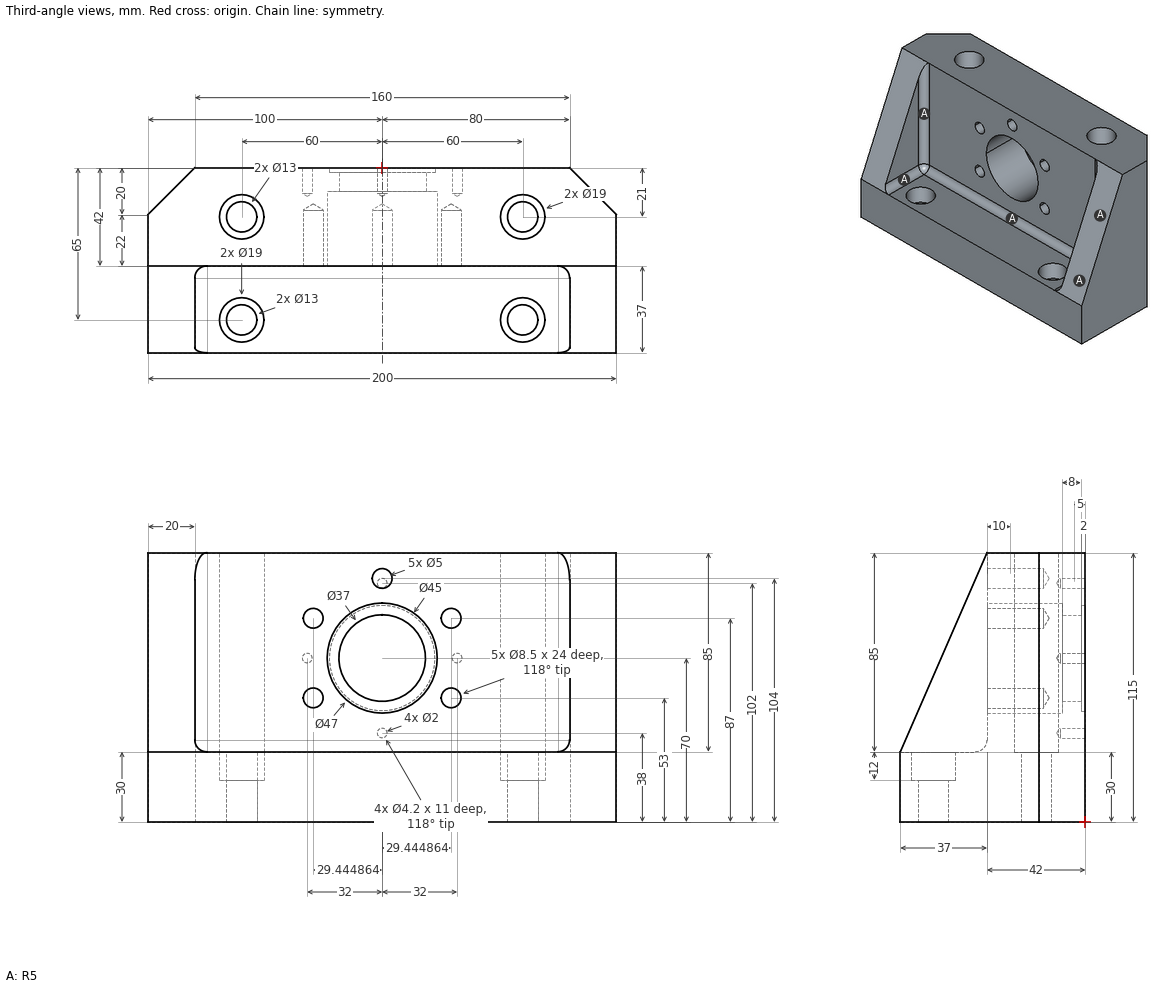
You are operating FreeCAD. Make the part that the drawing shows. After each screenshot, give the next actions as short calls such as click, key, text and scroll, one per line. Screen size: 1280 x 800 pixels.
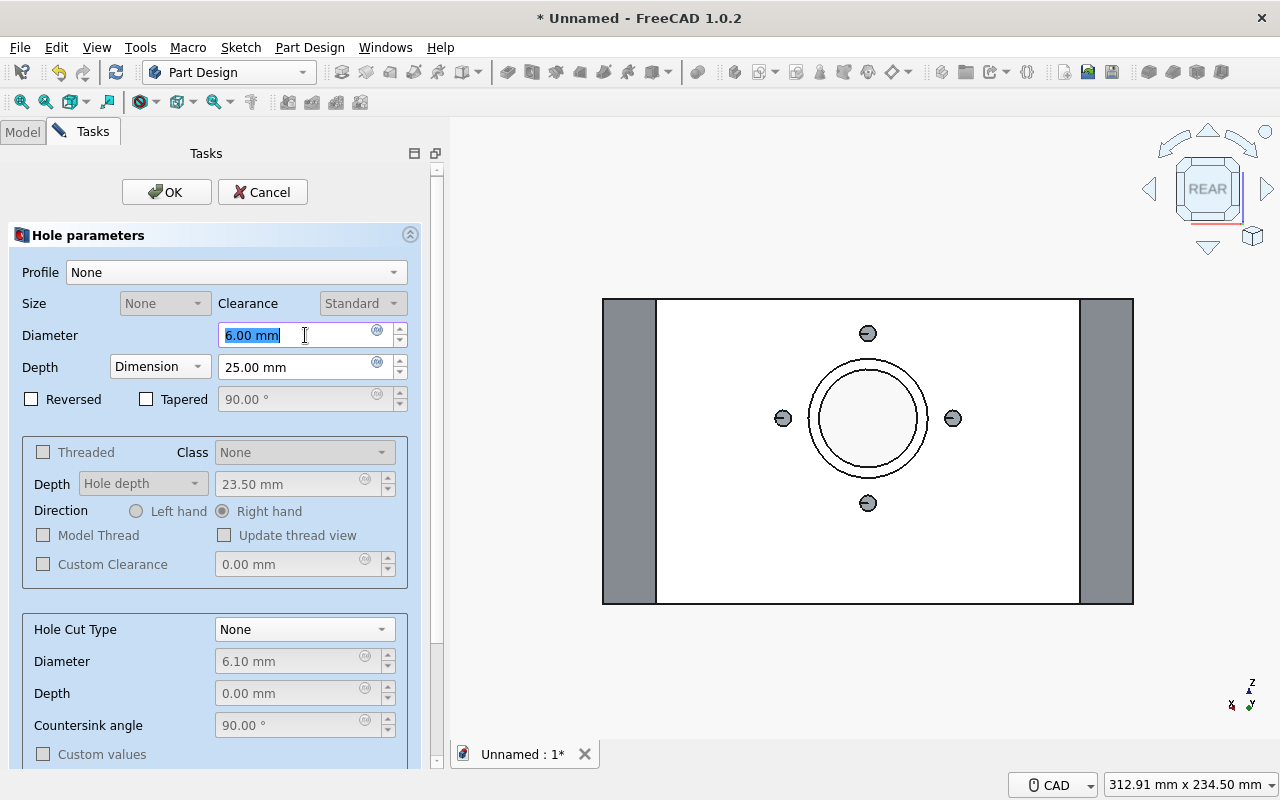
text(4.2)
key(Tab)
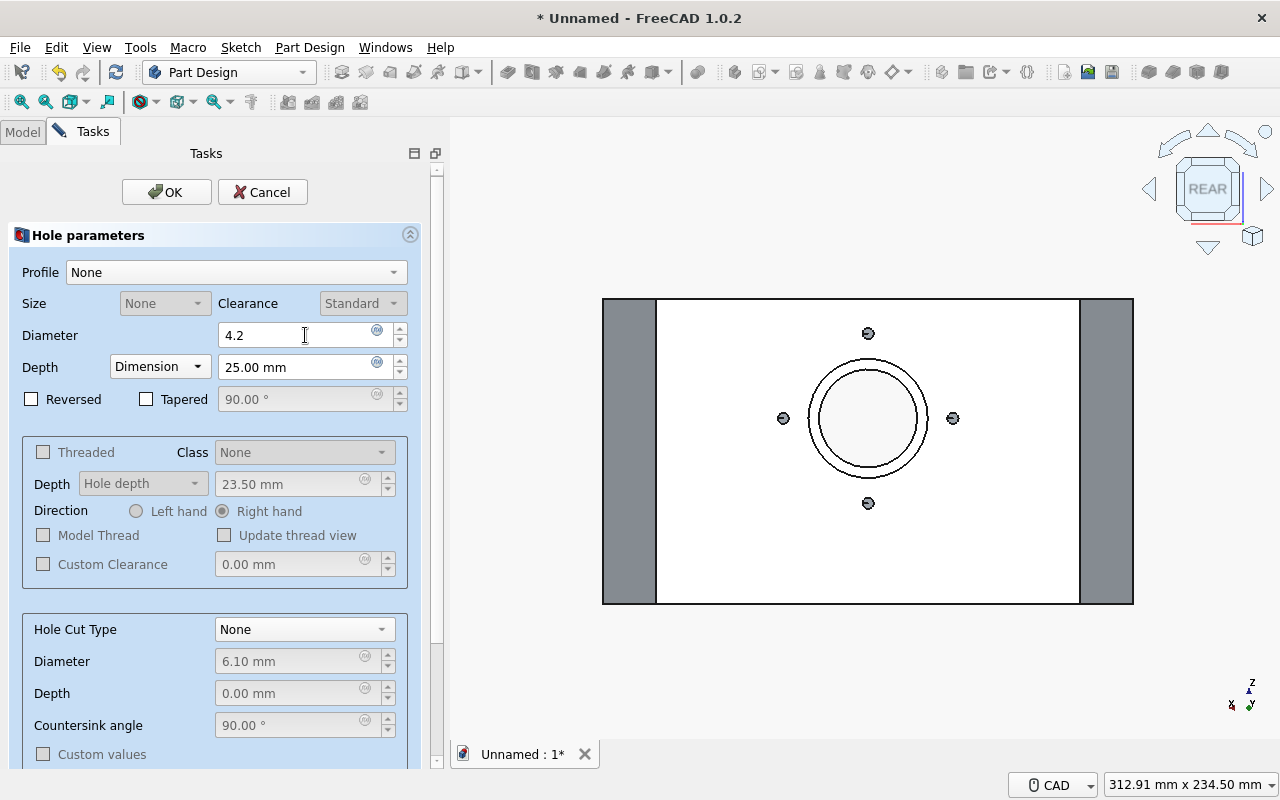
triple_click(305, 367)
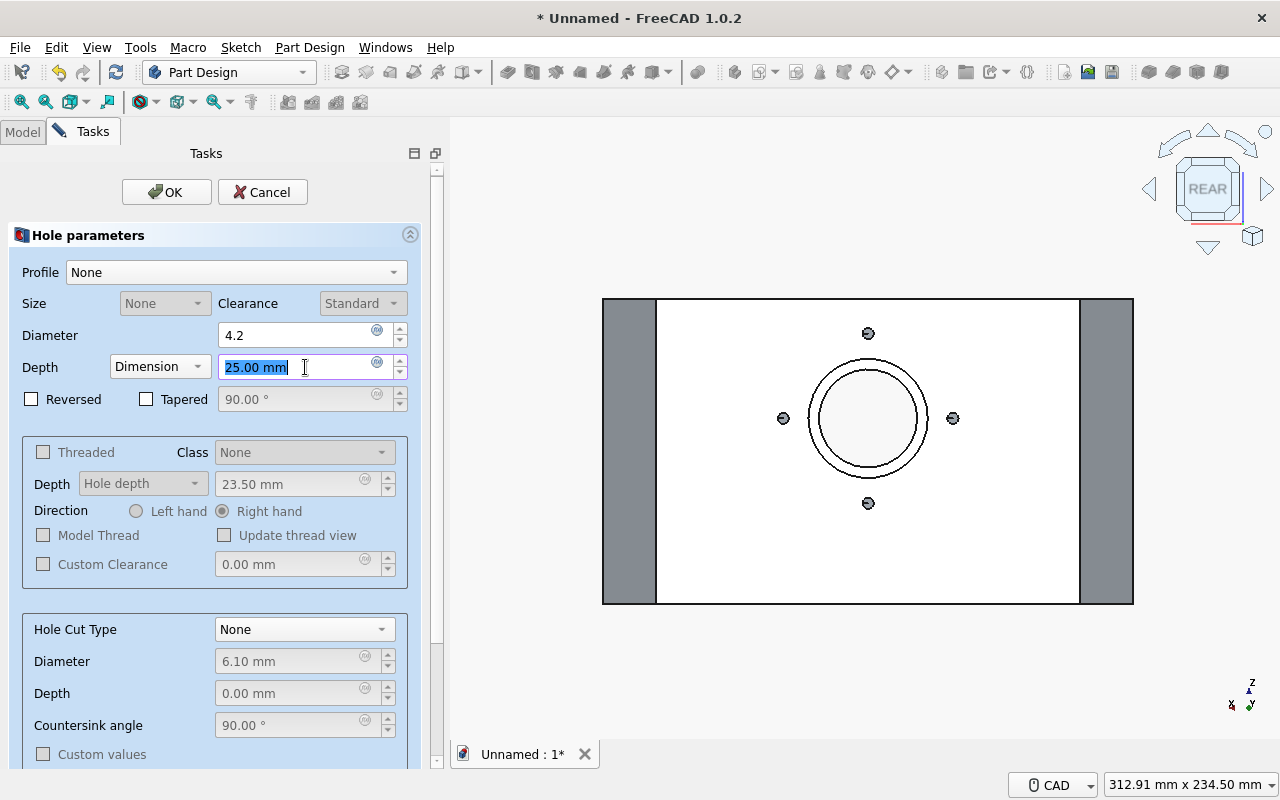
text(11)
key(Tab)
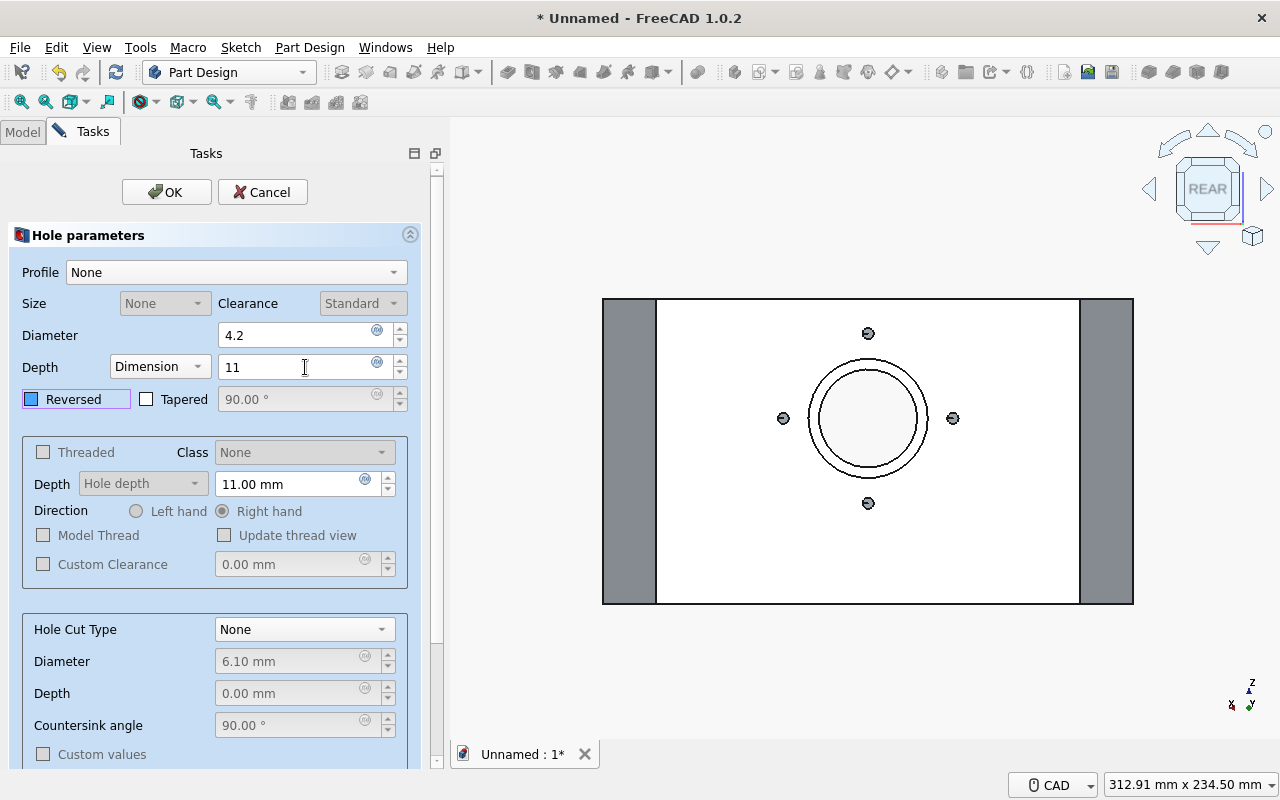
click(167, 192)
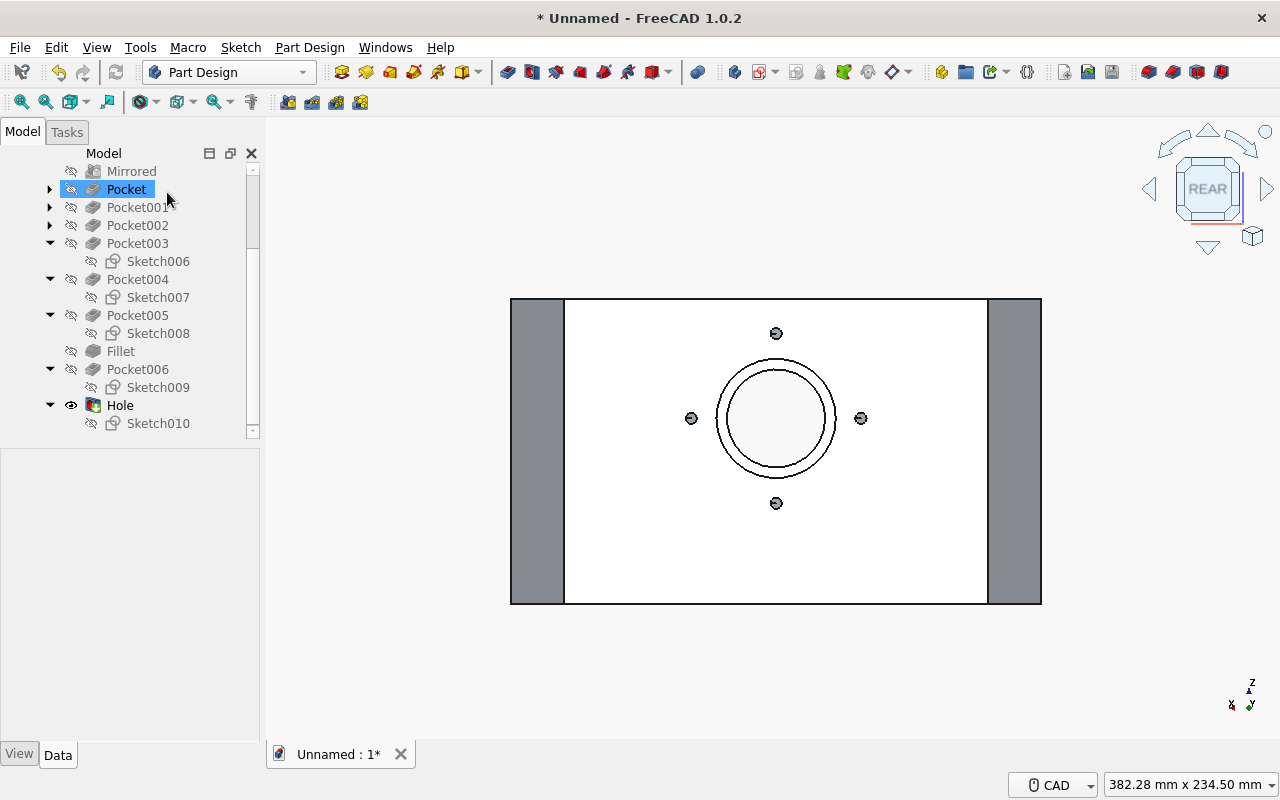
key(0)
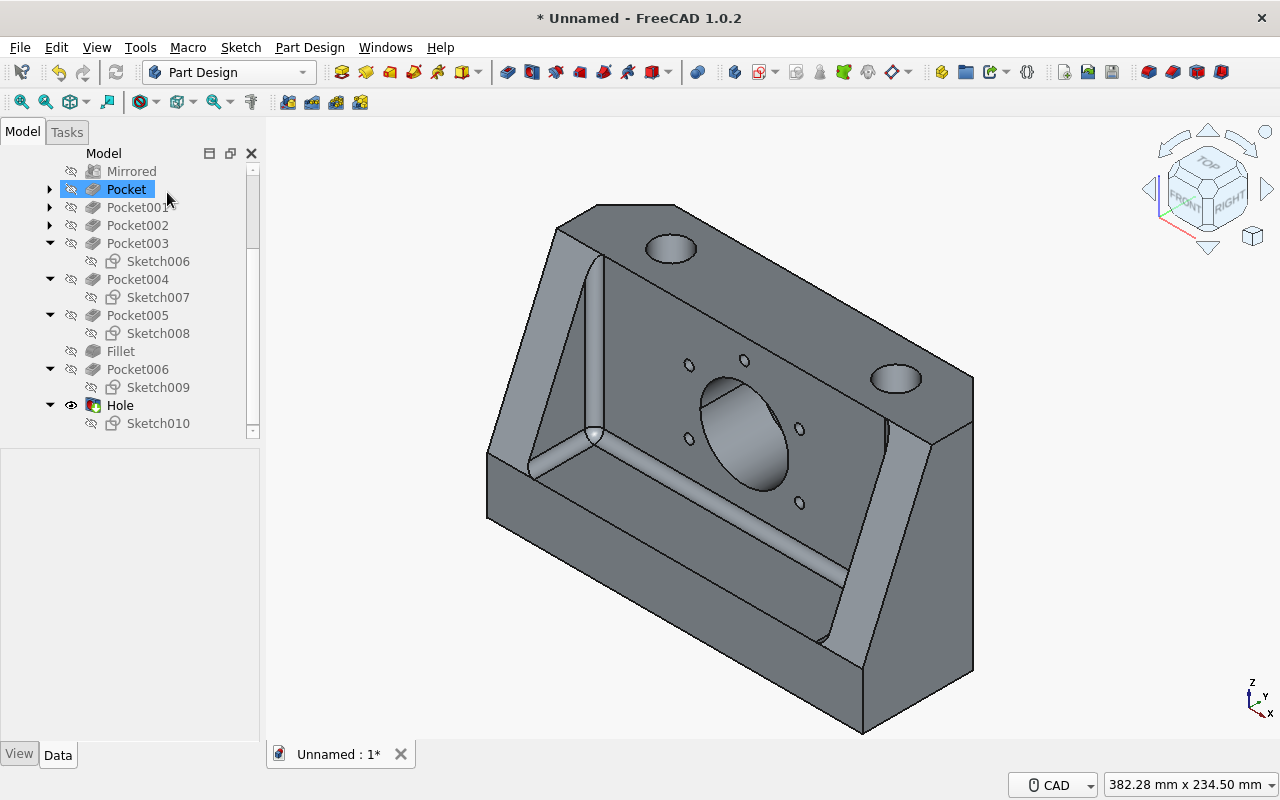
click(825, 469)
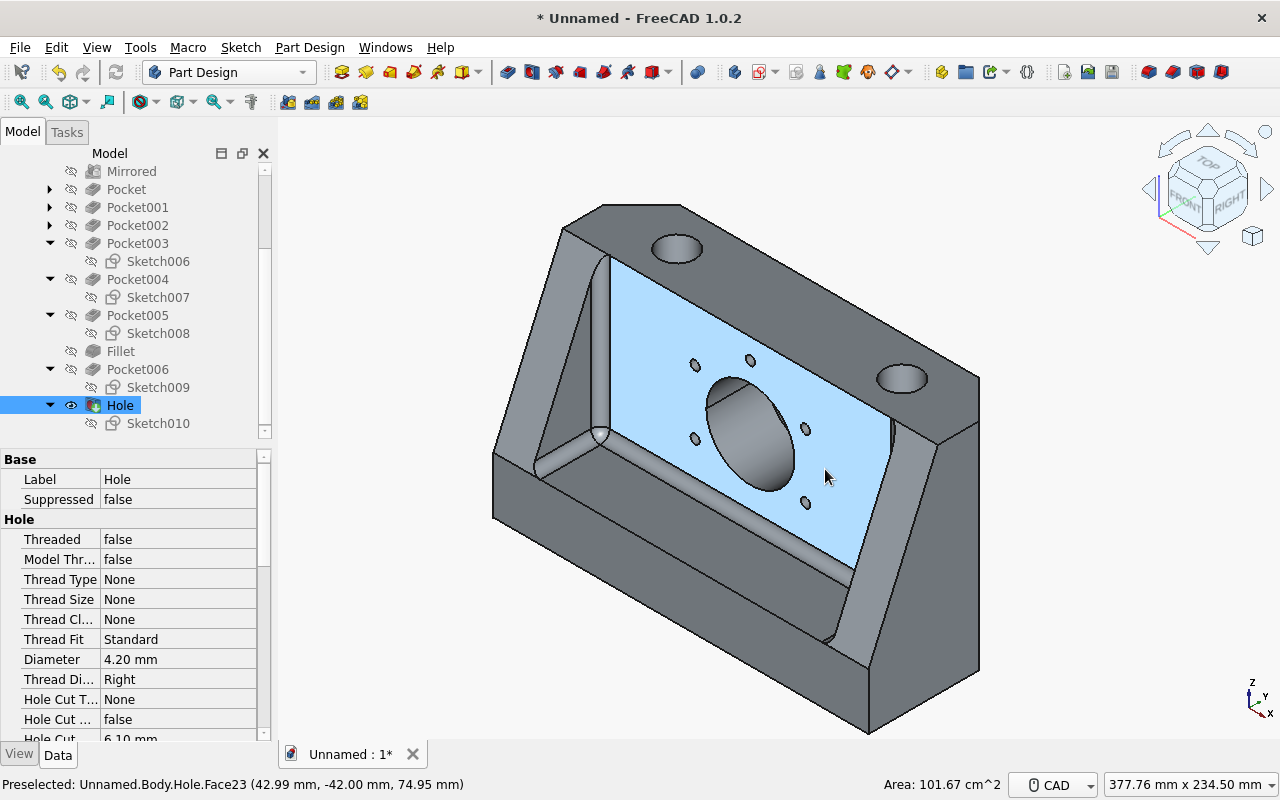
click(760, 72)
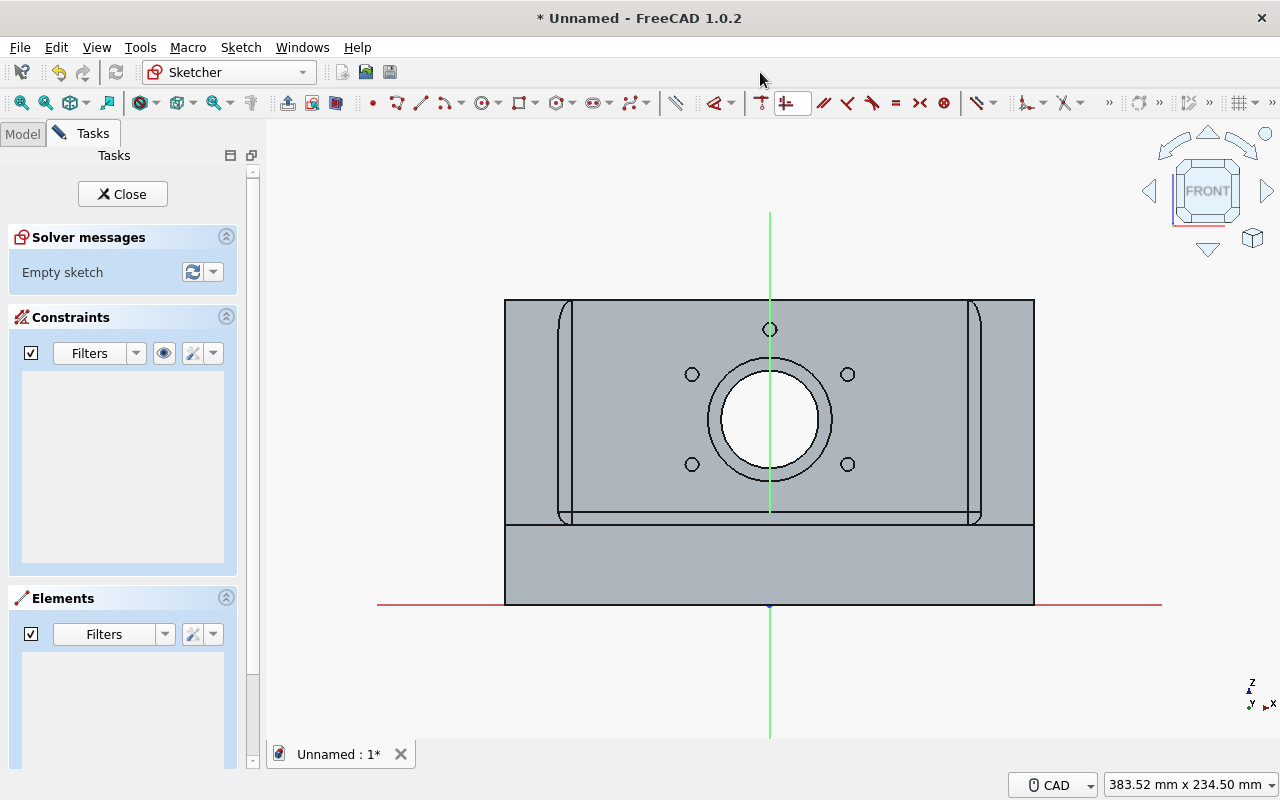
scroll(903, 527, up, 2)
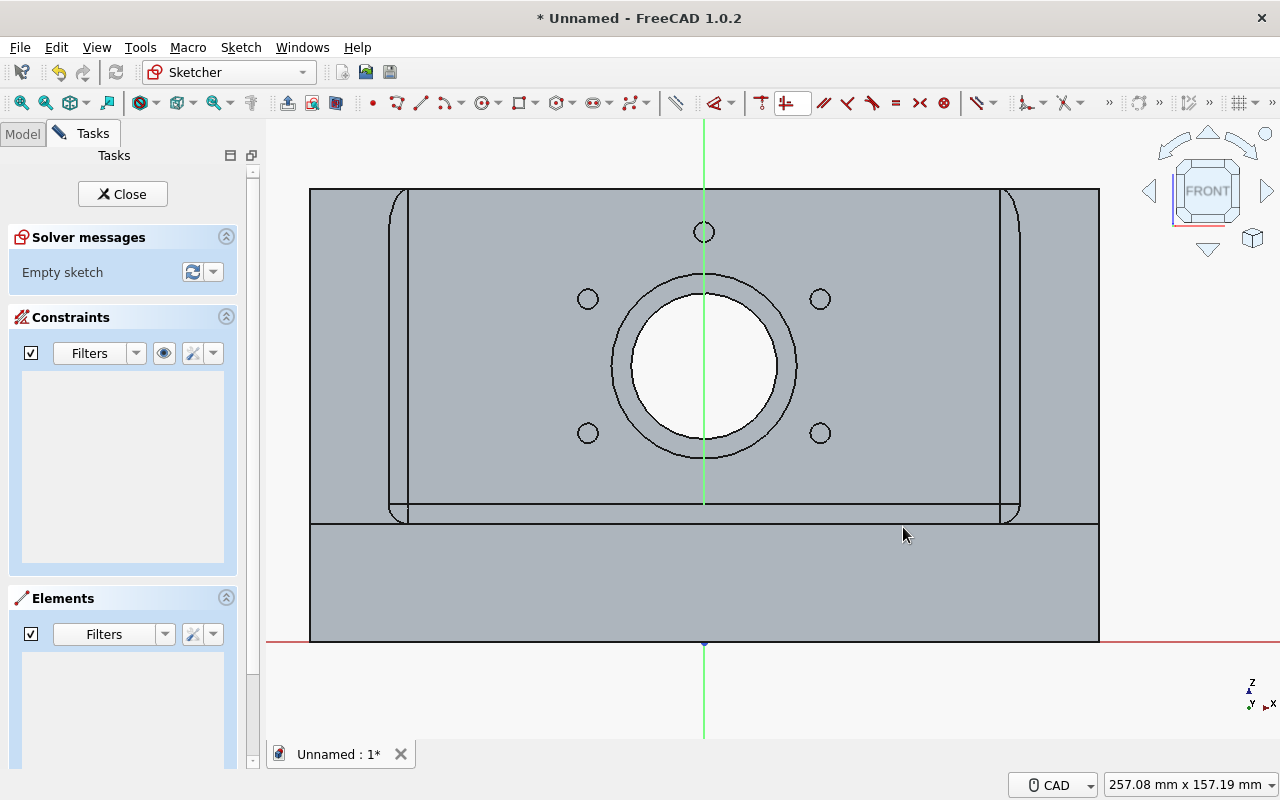
click(482, 104)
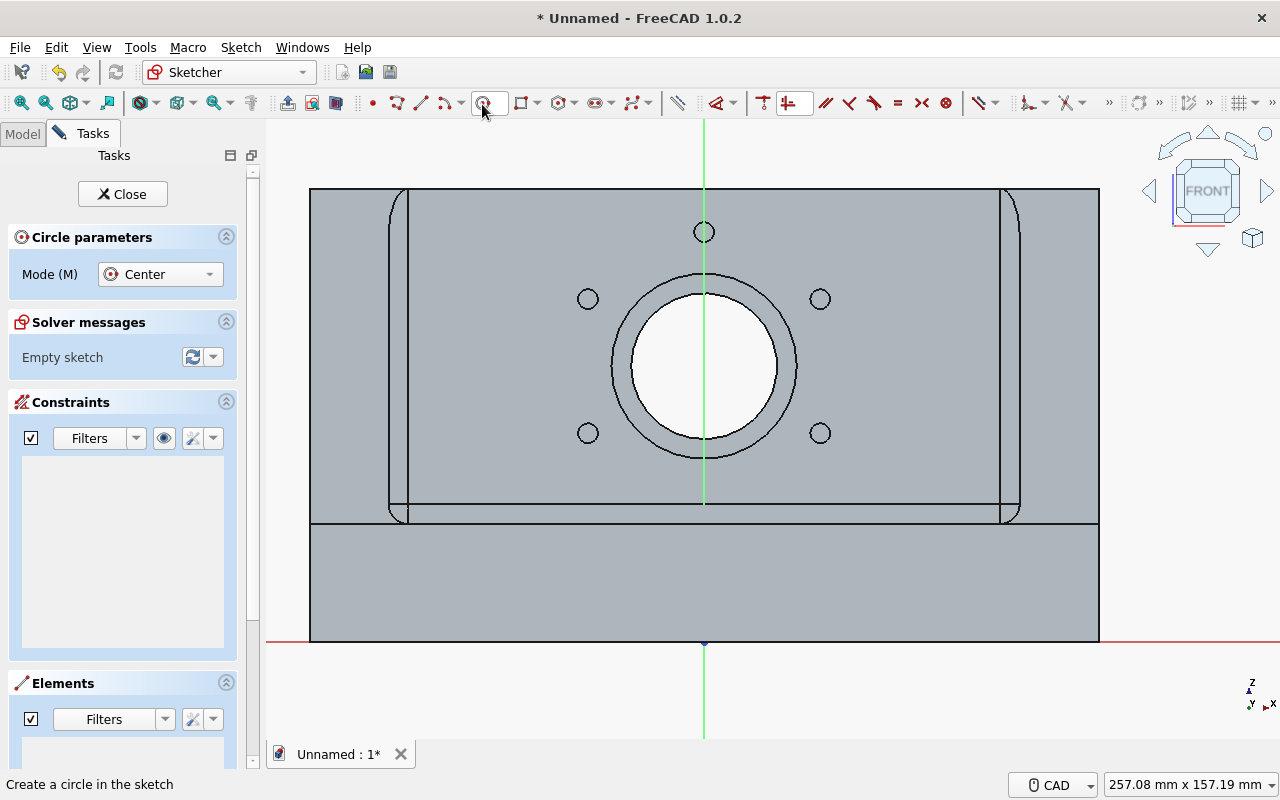
scroll(820, 433, up, 2)